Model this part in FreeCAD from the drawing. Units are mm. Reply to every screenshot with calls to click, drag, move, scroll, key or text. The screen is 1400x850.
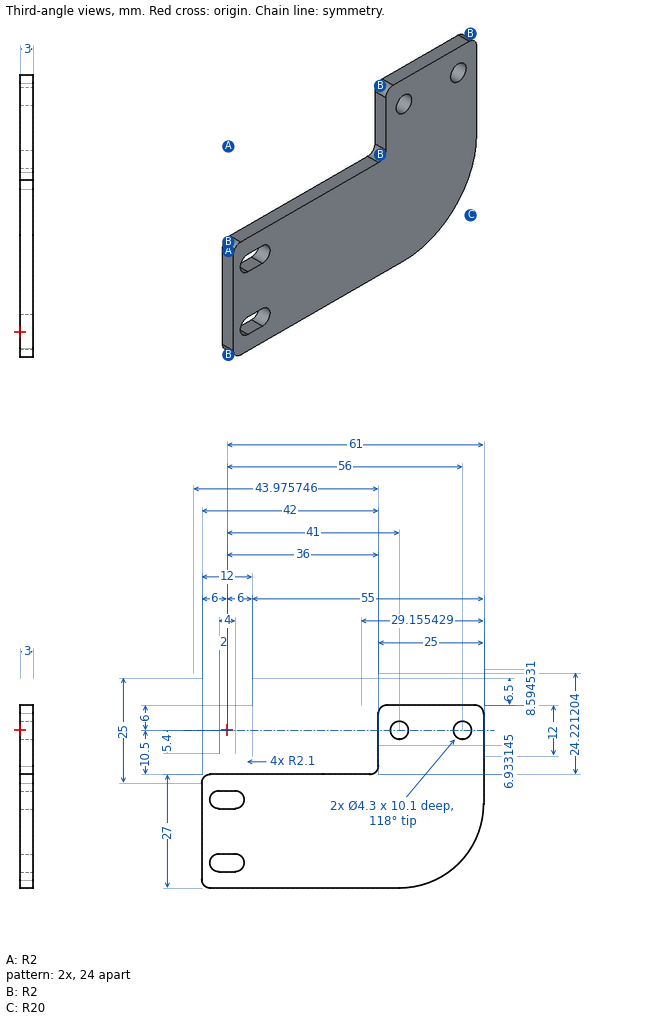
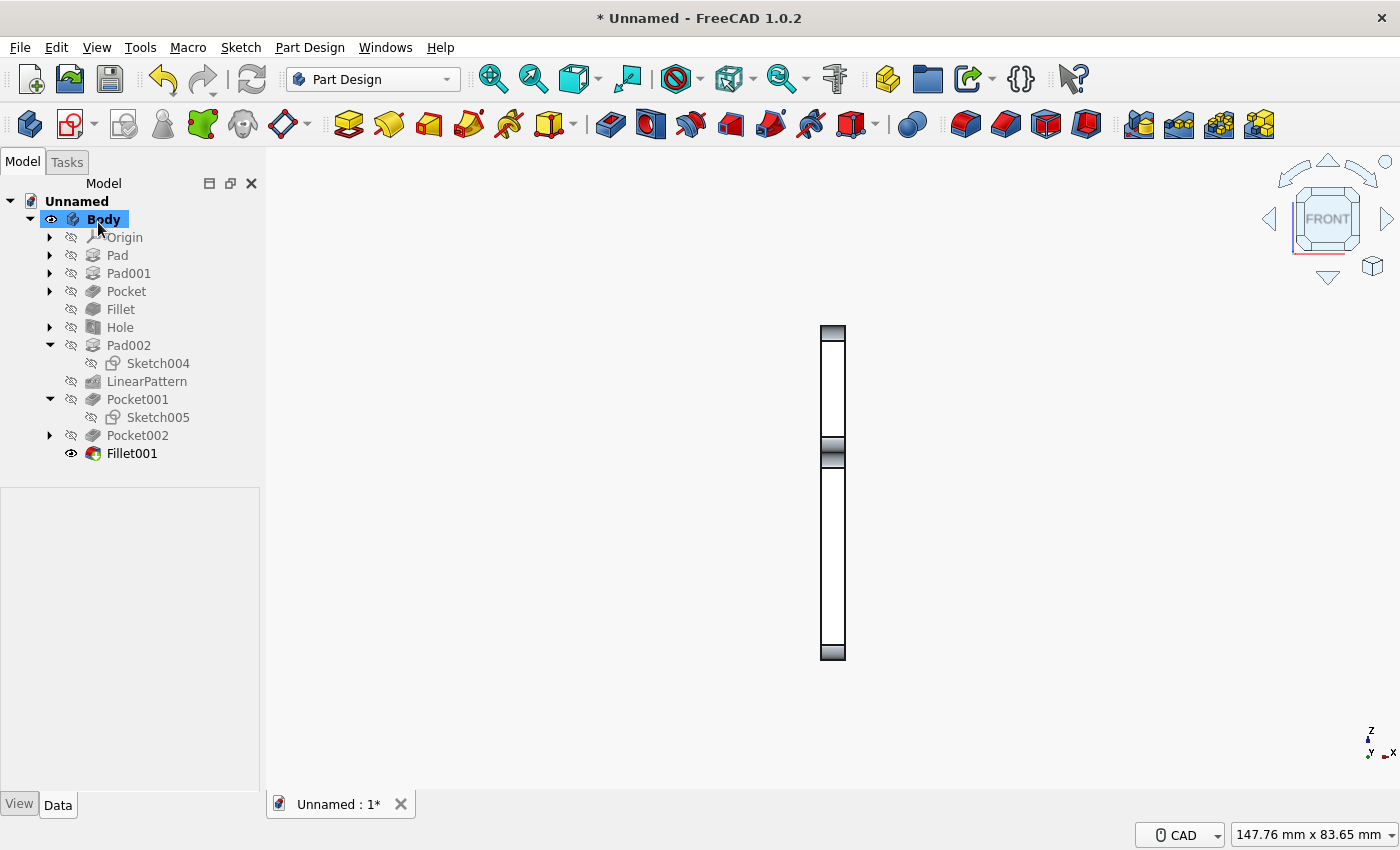
key(3)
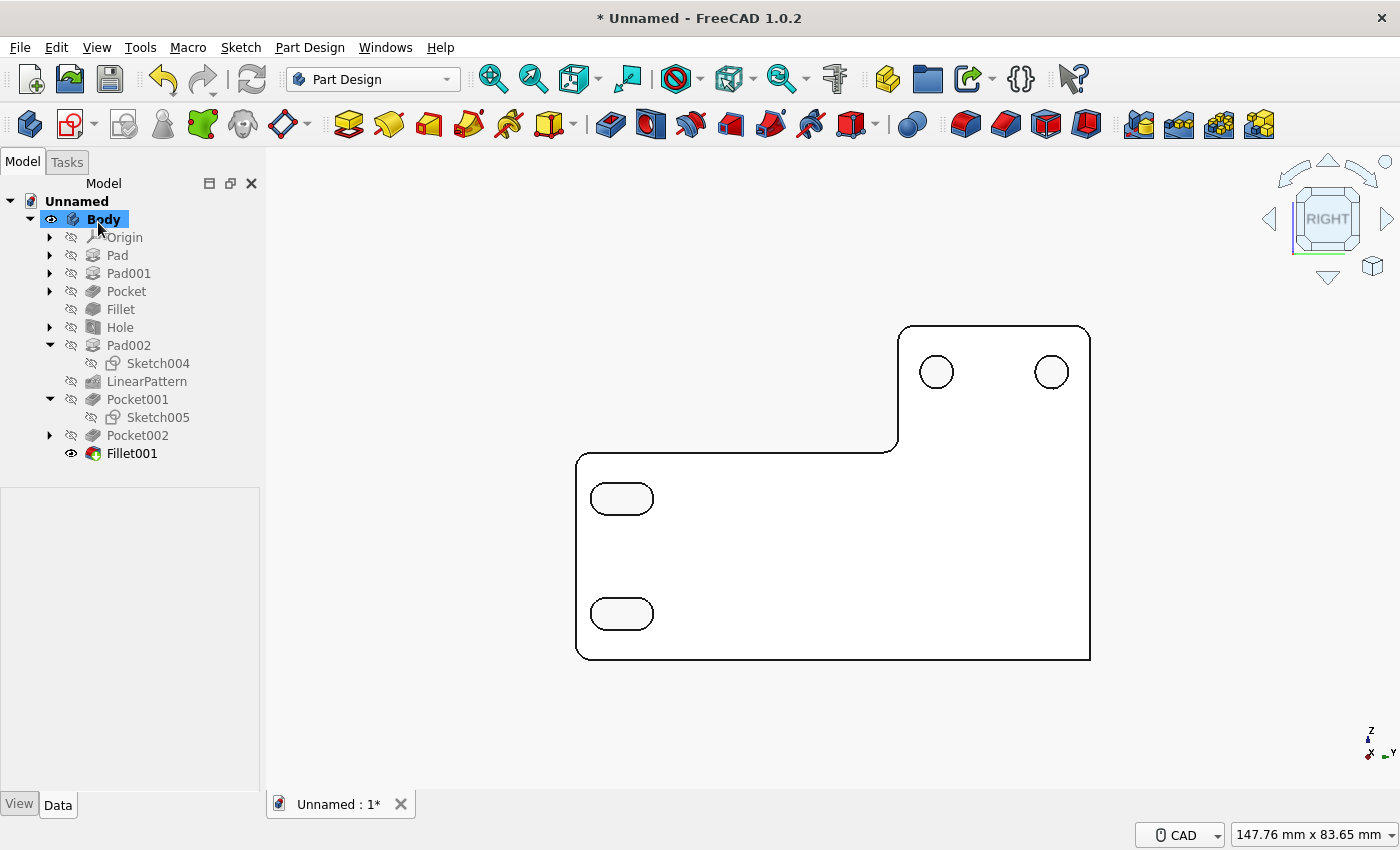
key(5)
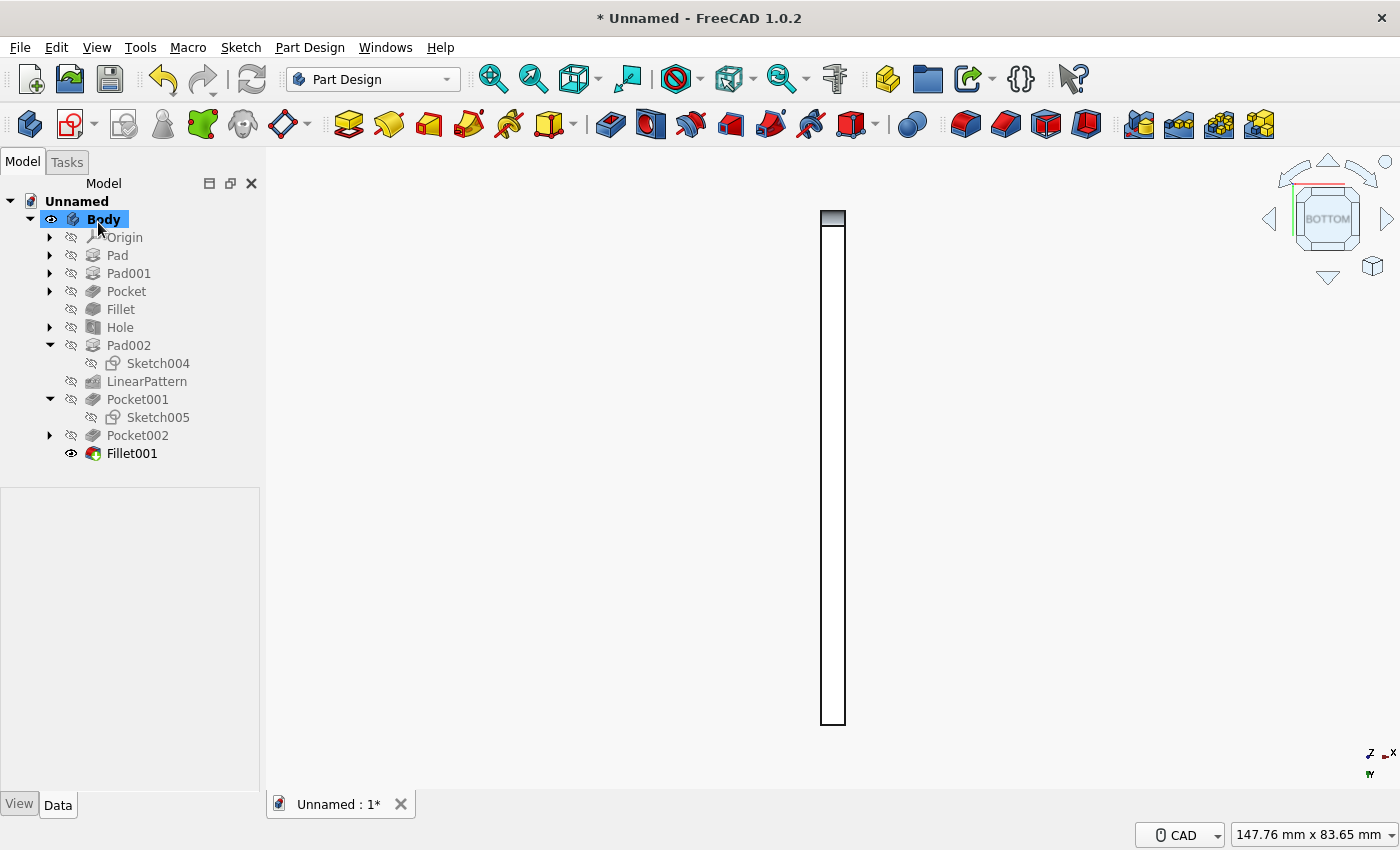
click(833, 724)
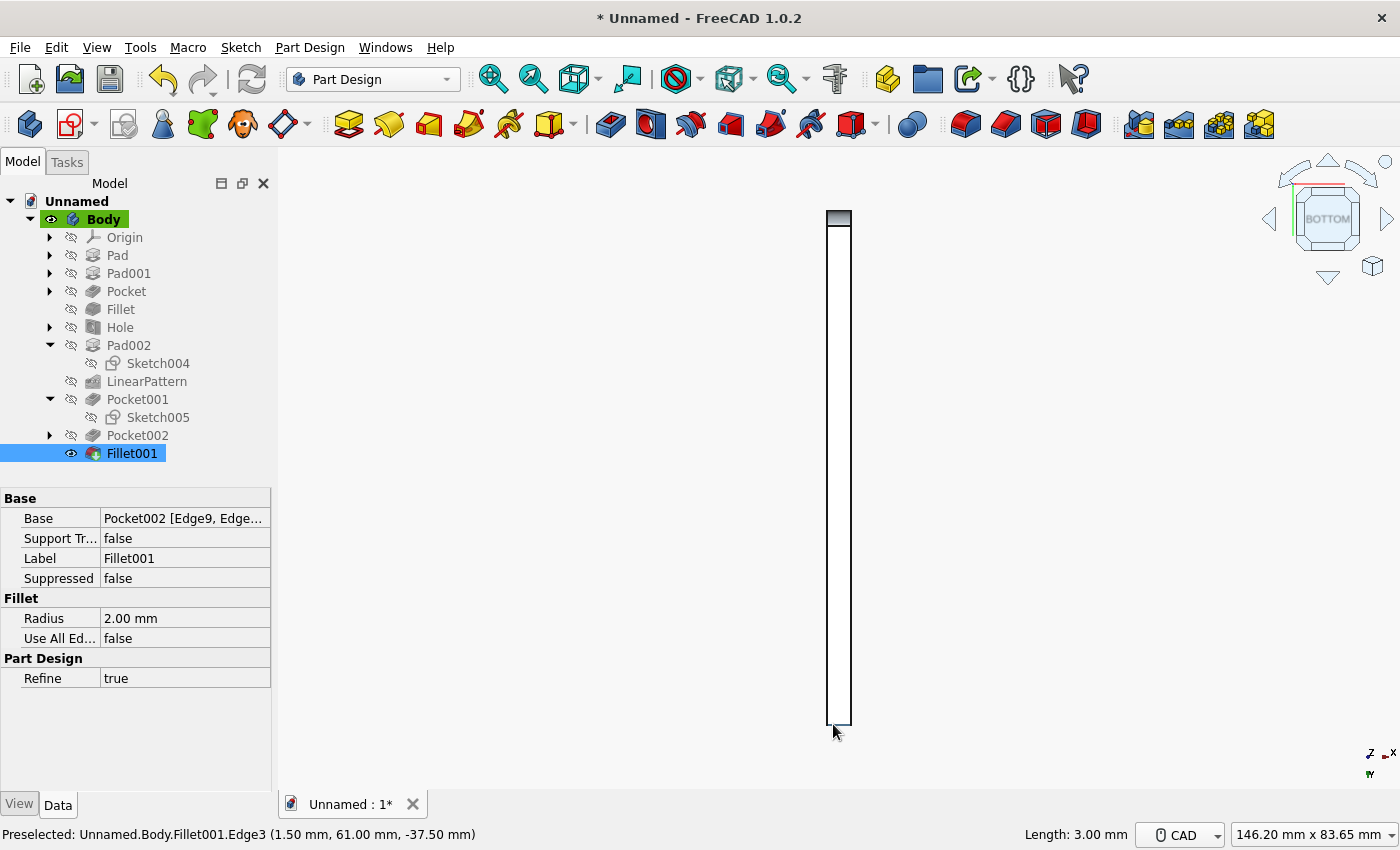
click(966, 124)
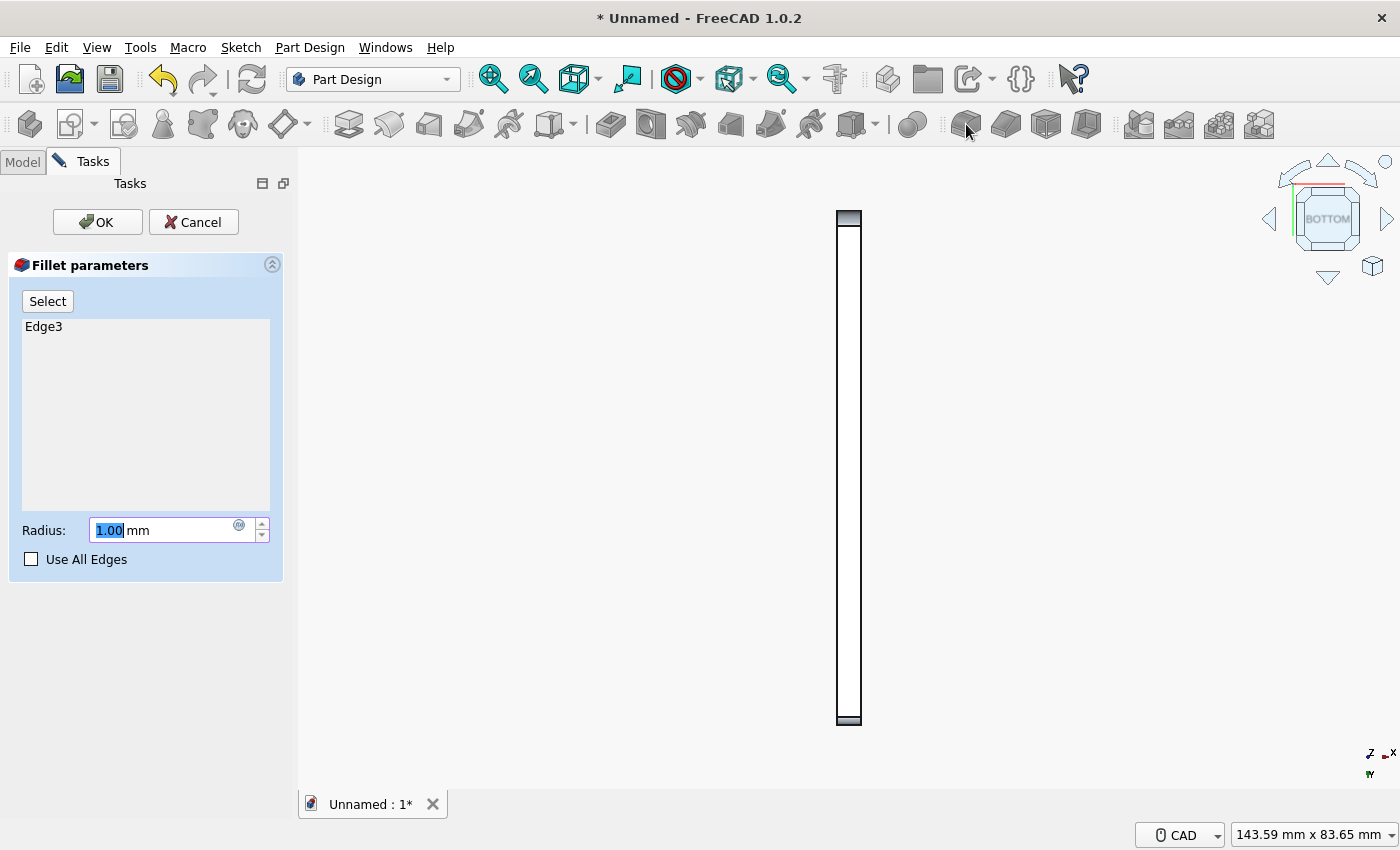
text(20)
key(Tab)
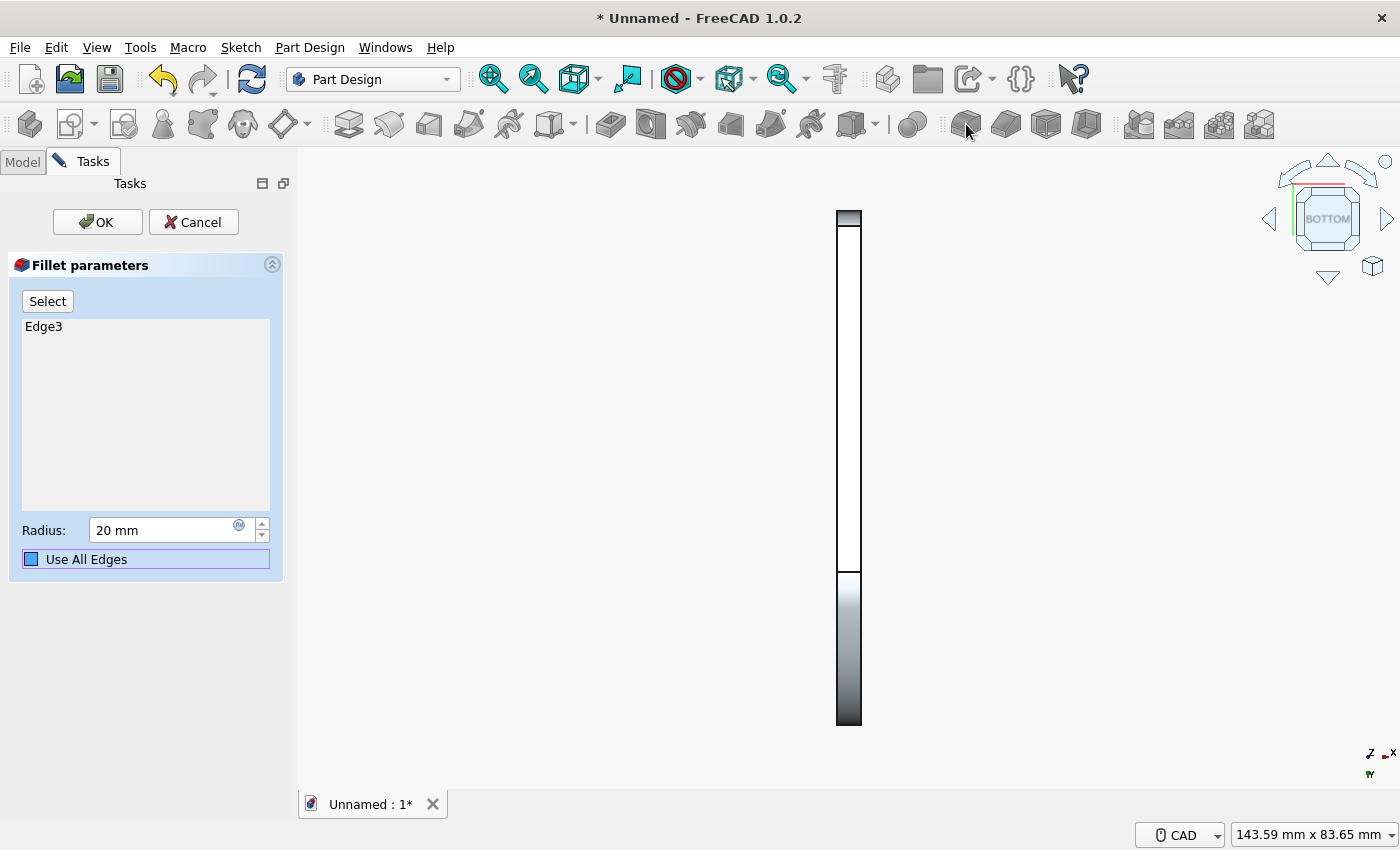
click(98, 222)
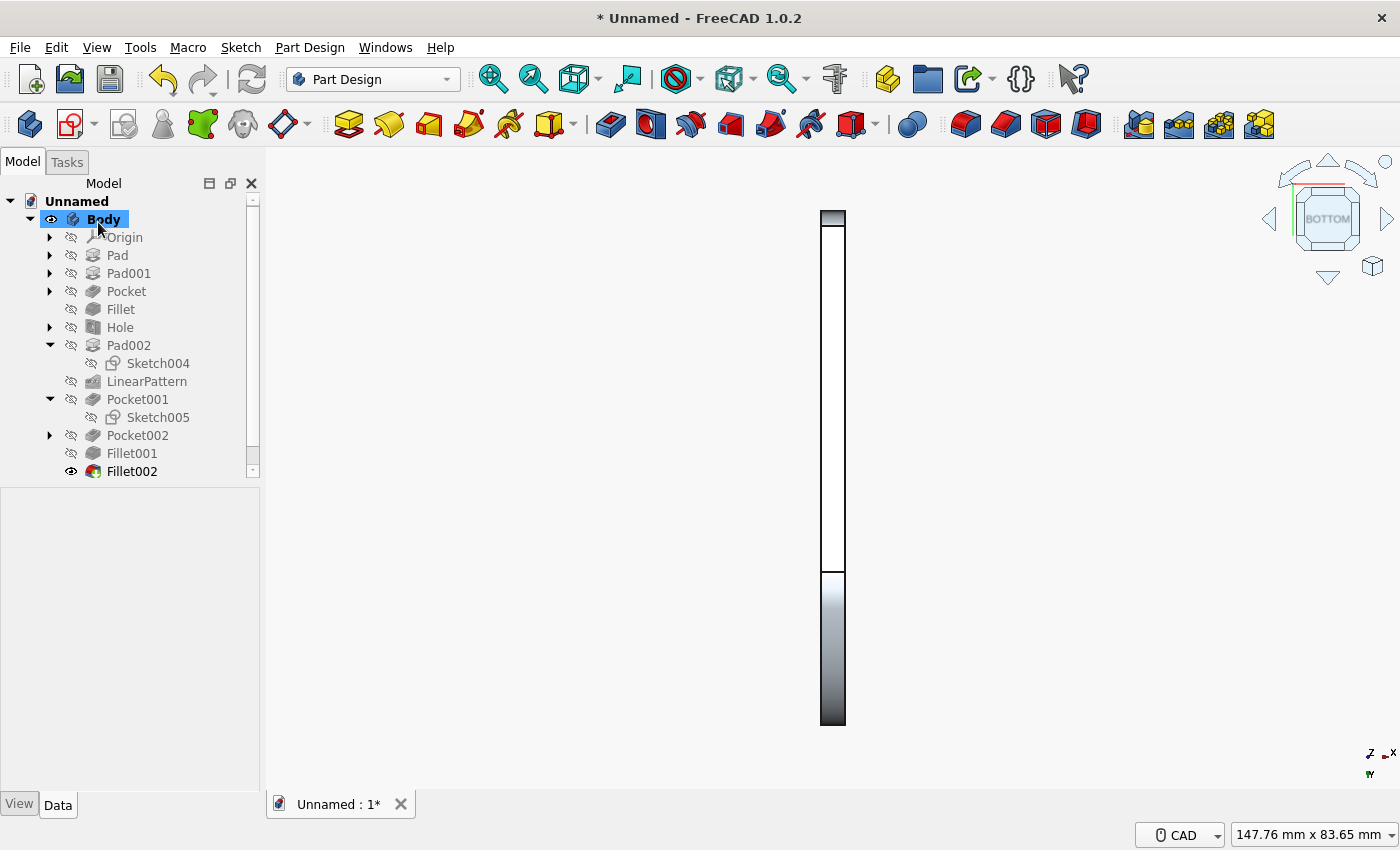
key(0)